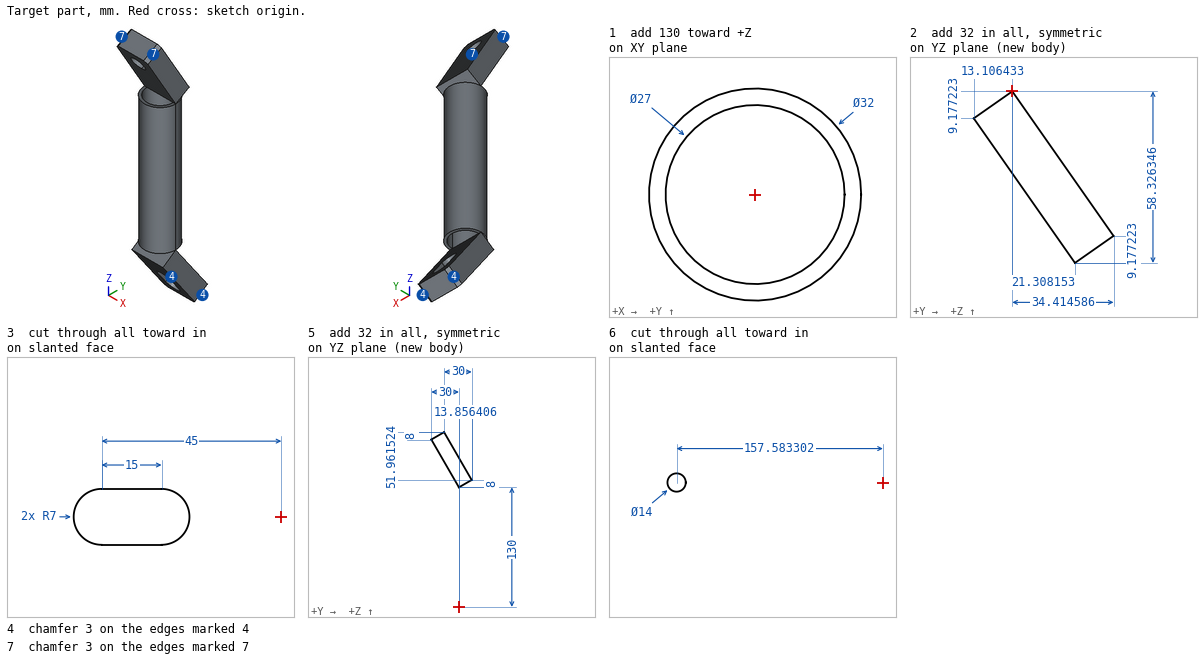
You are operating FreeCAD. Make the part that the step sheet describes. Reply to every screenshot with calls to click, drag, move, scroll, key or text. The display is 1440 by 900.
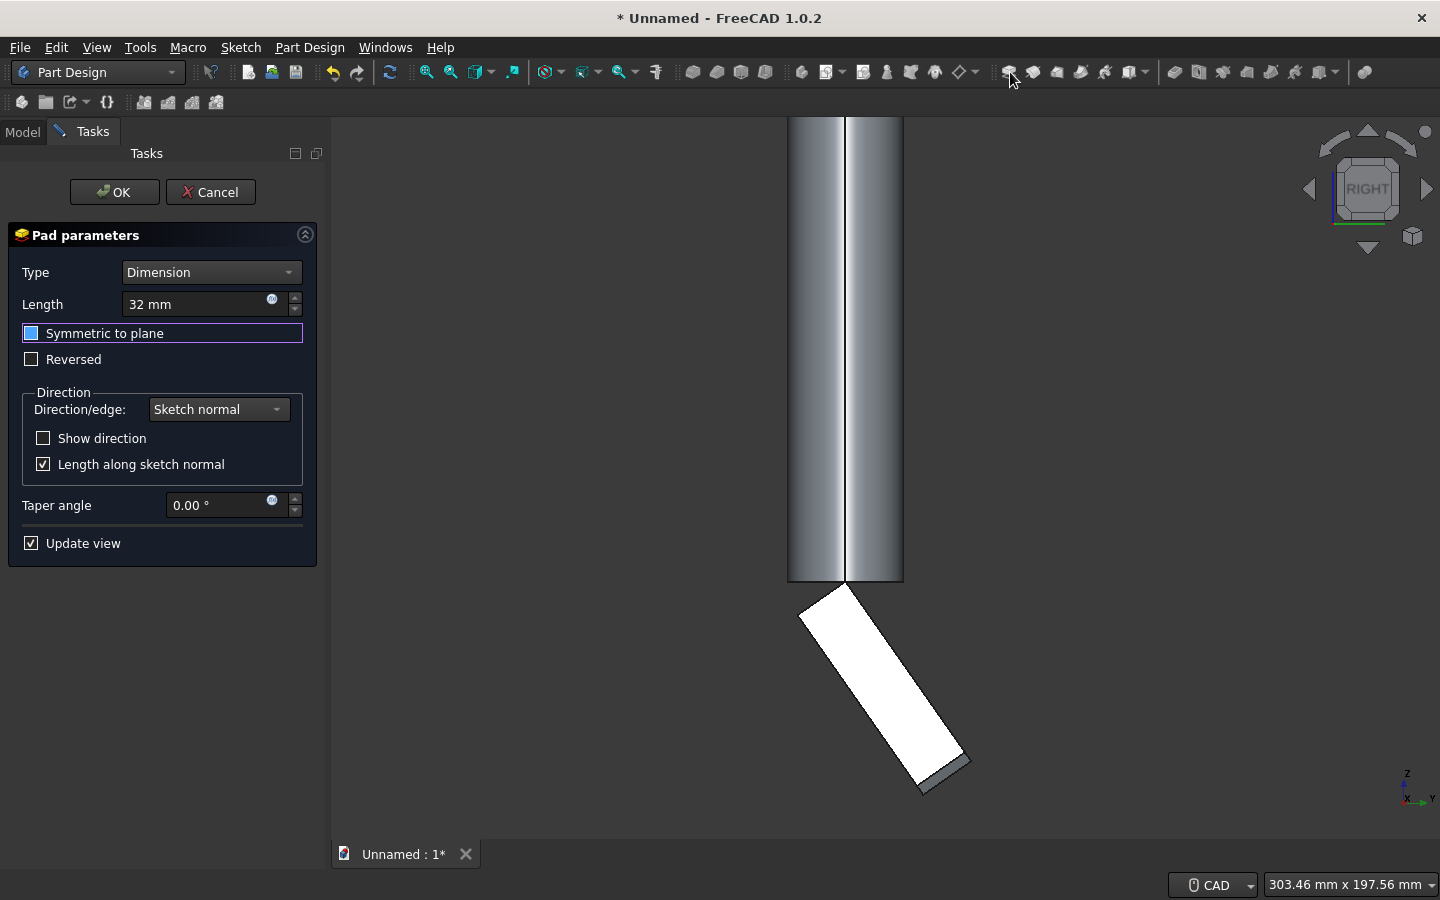
click(30, 333)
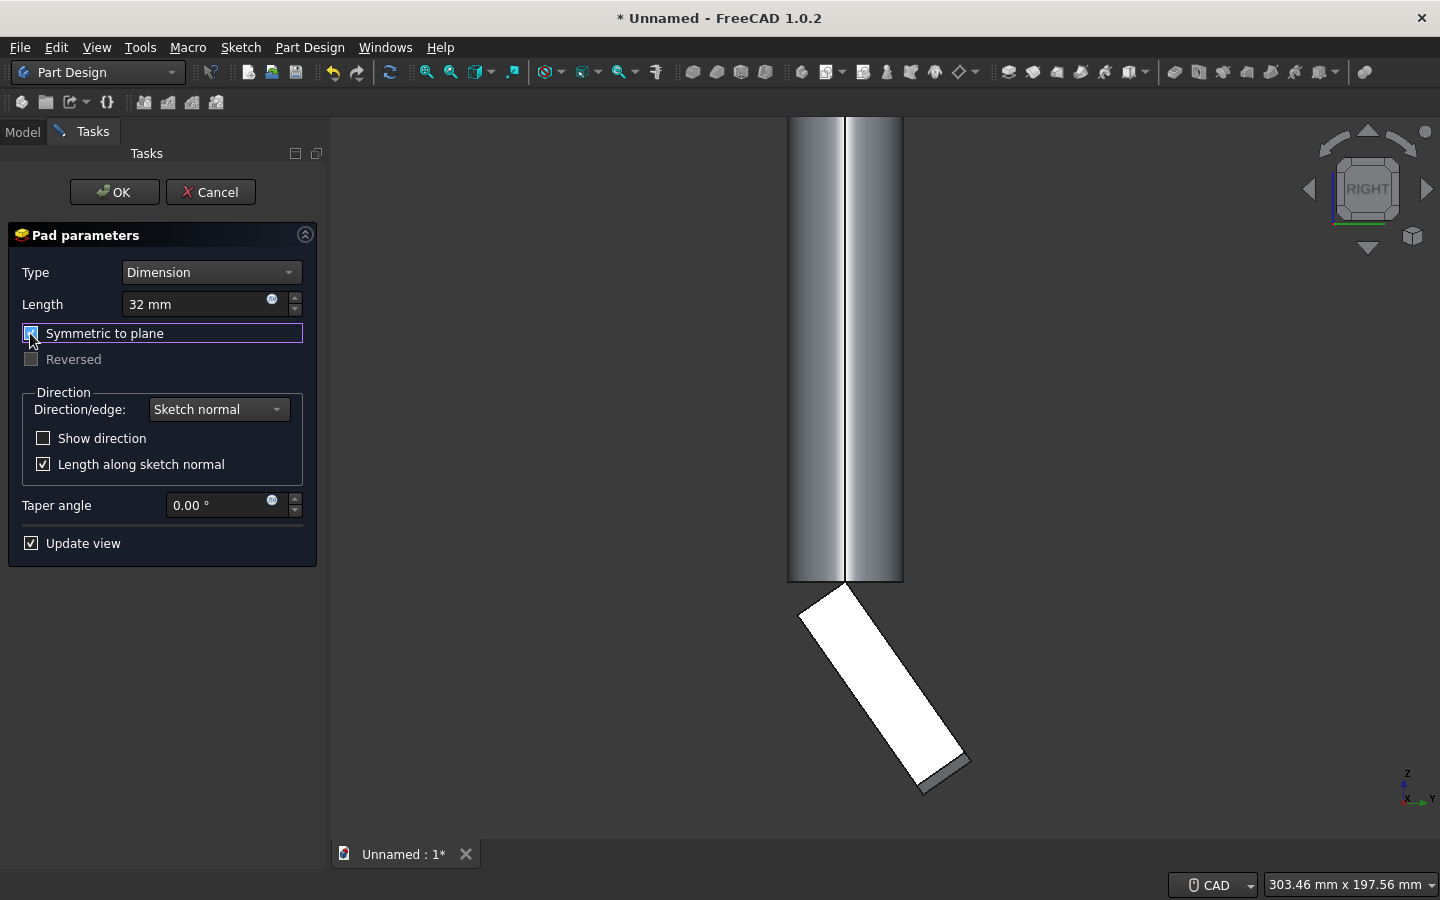
click(115, 192)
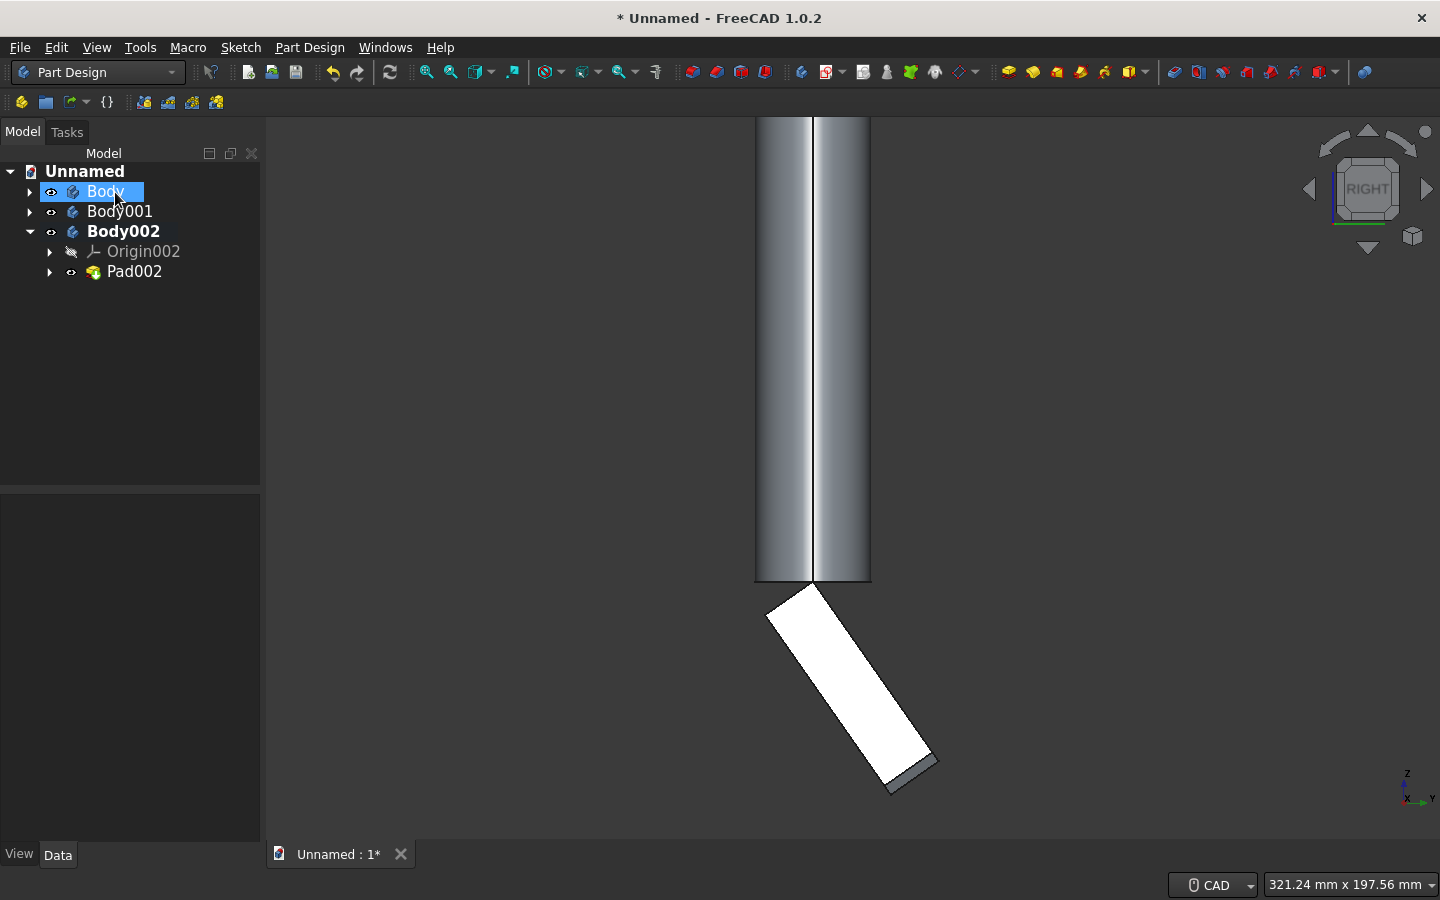
key(v)
key(f)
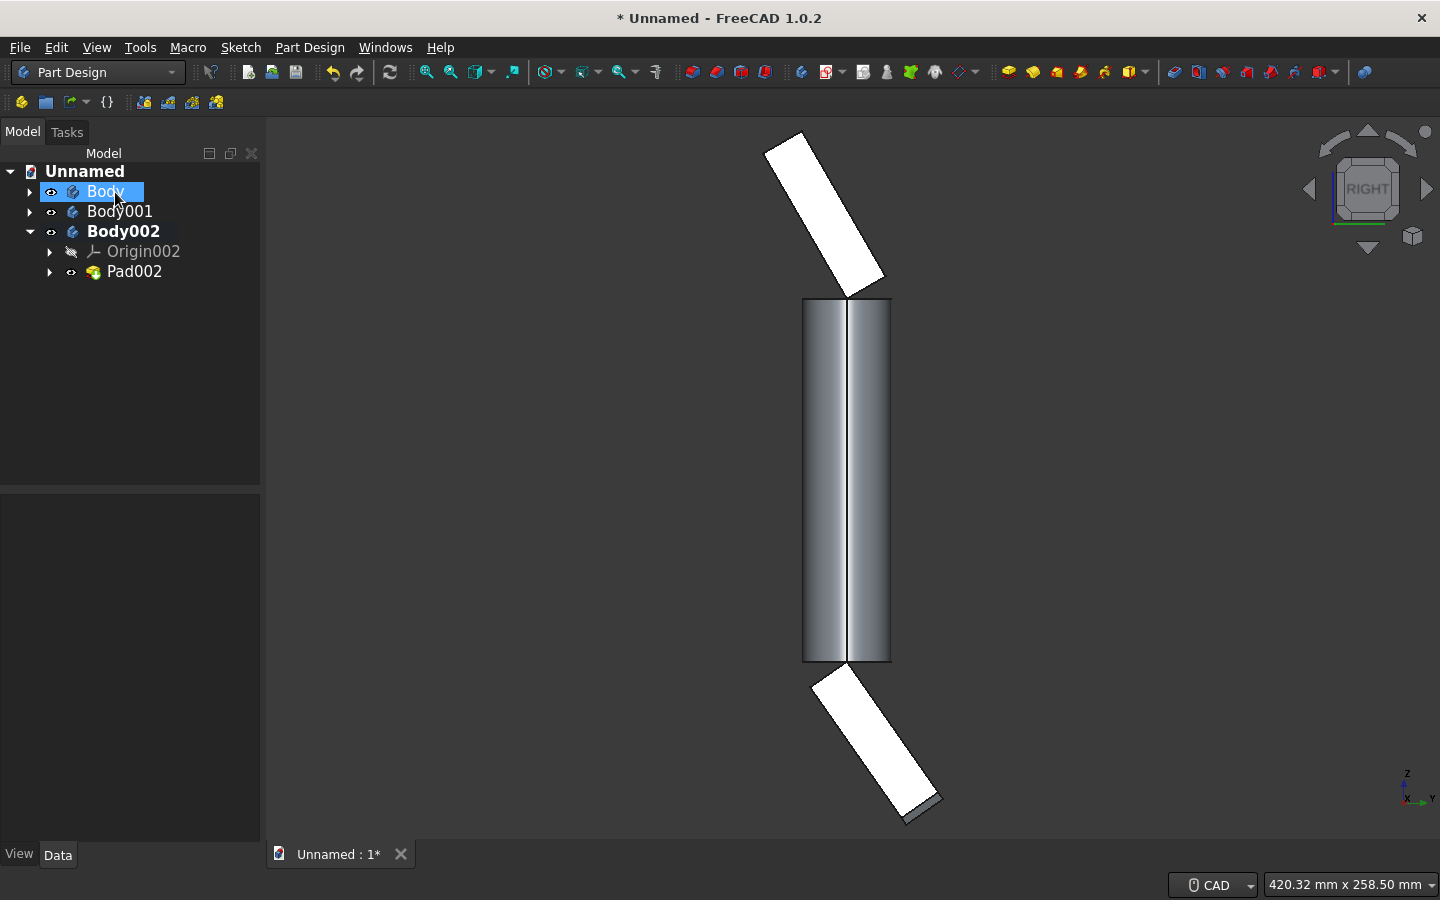
key(1)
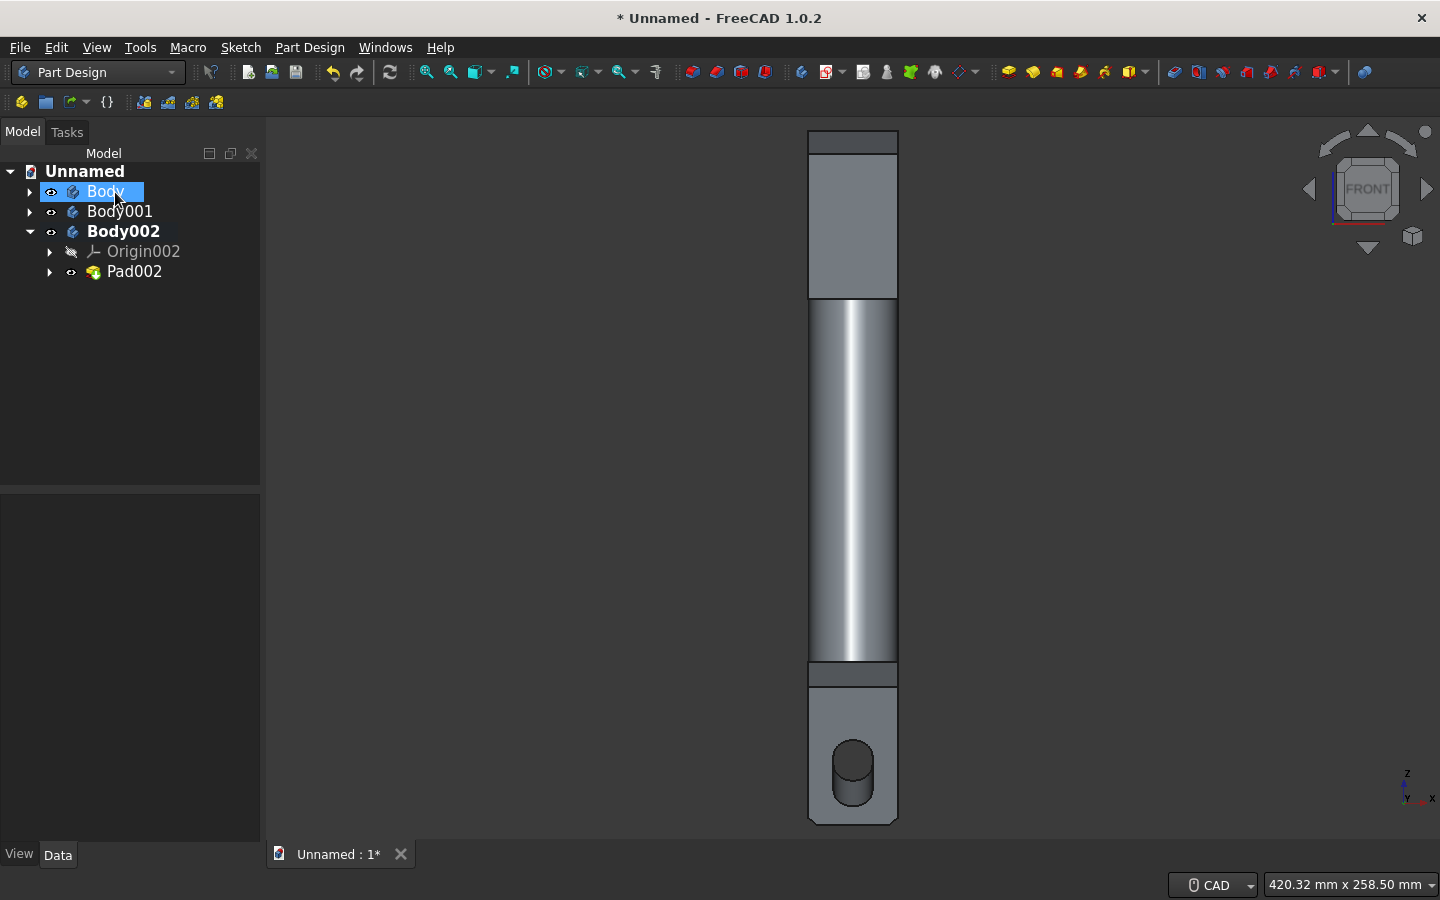
click(428, 72)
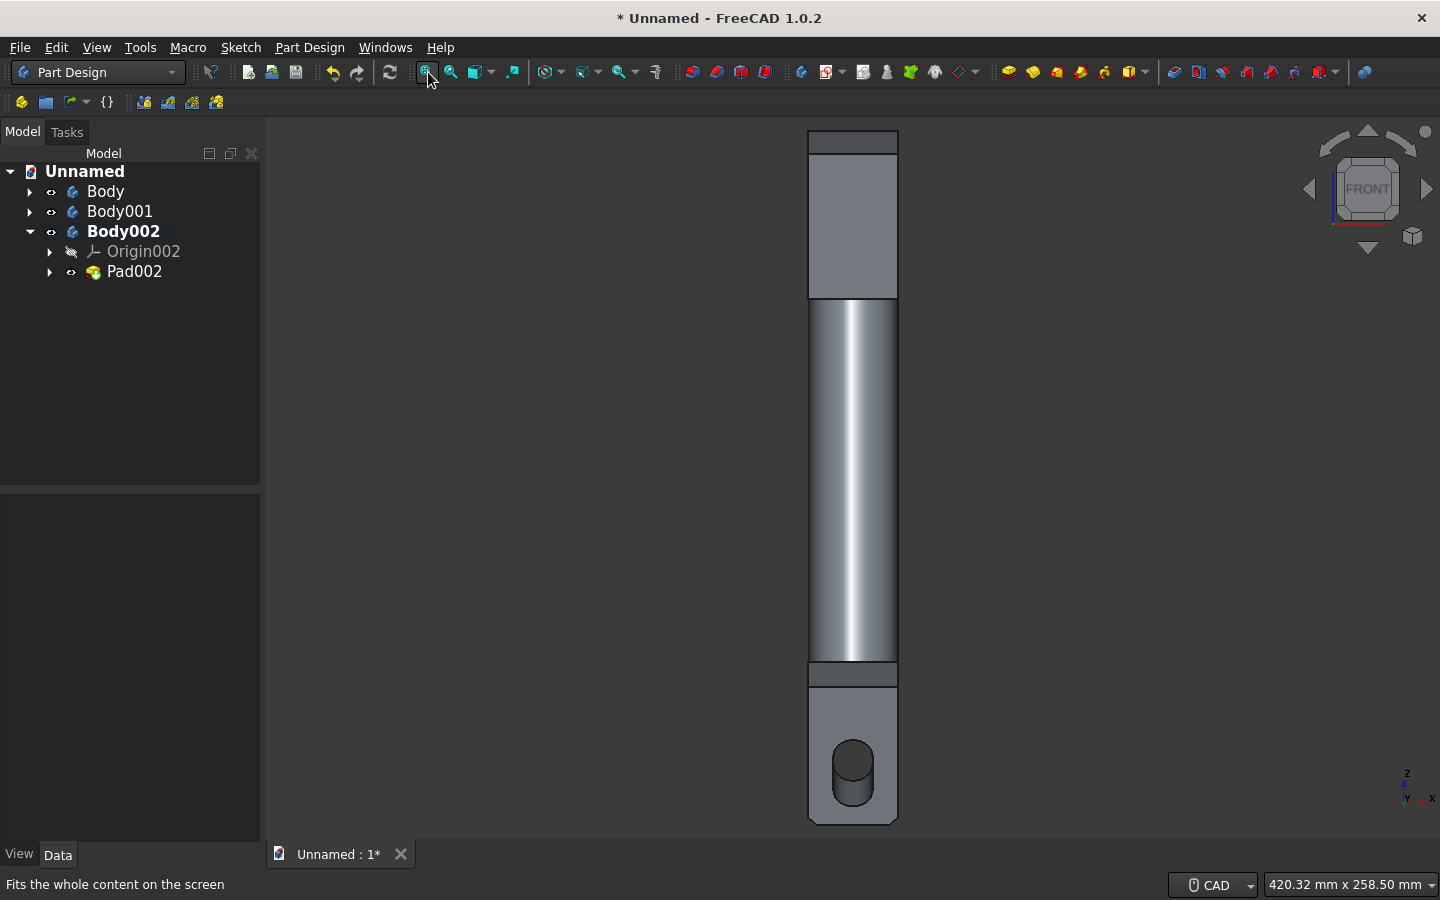
click(853, 246)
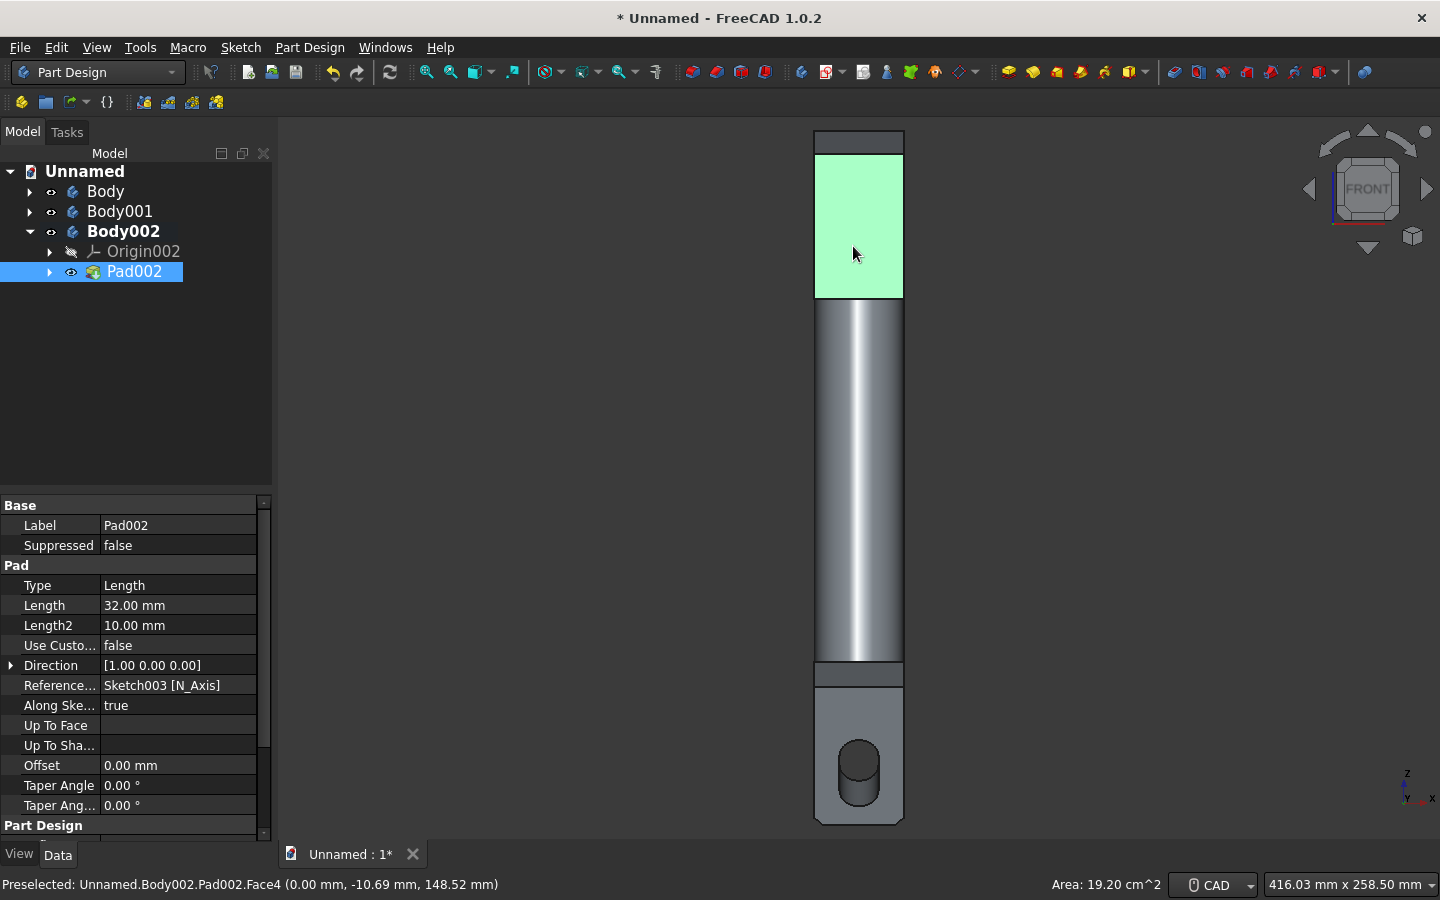
click(826, 72)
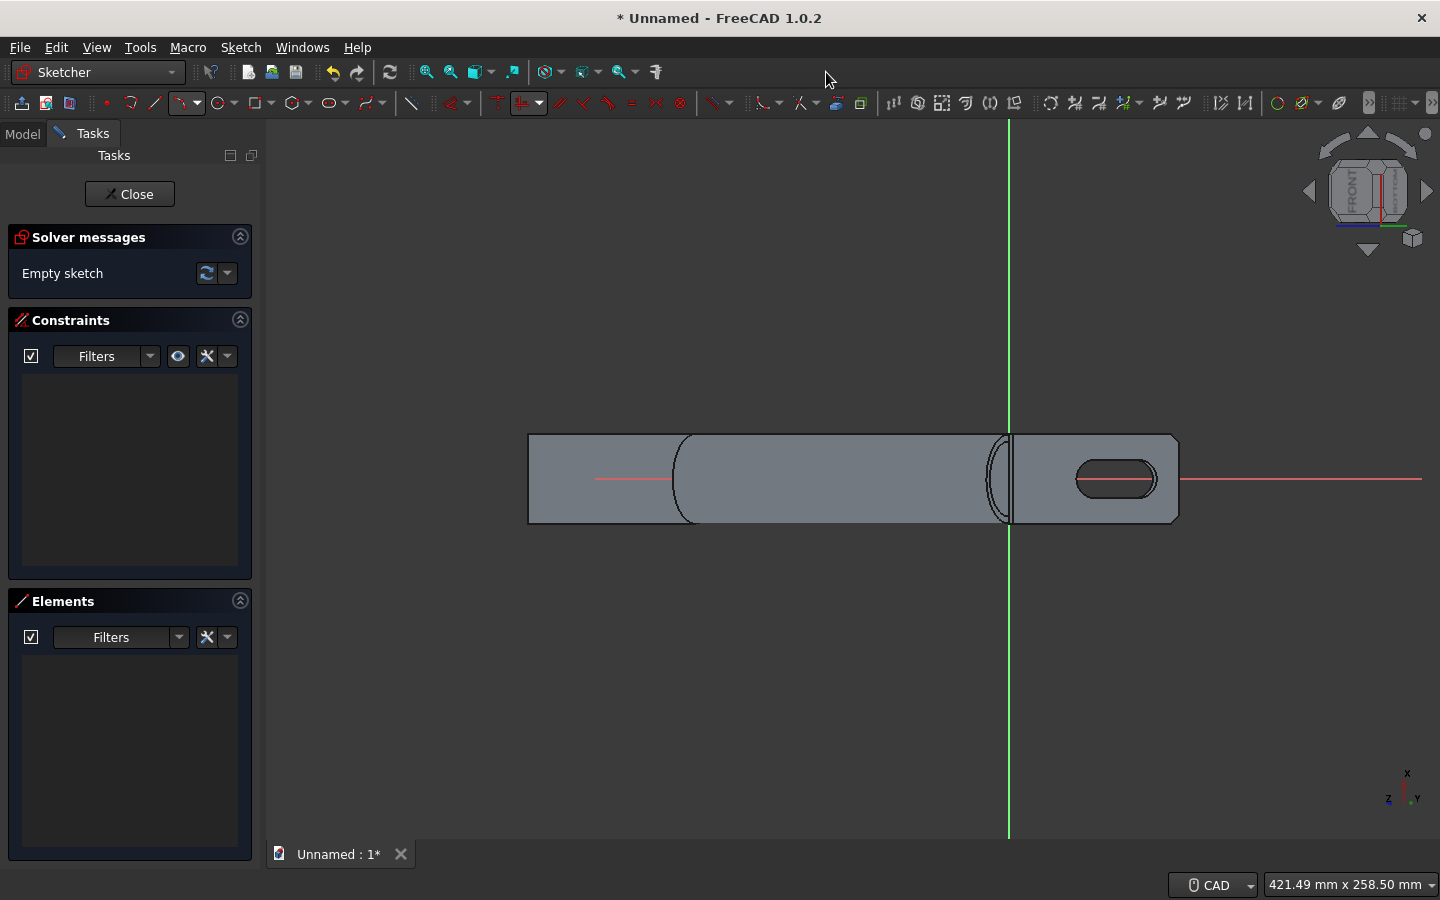
key(q)
key(s)